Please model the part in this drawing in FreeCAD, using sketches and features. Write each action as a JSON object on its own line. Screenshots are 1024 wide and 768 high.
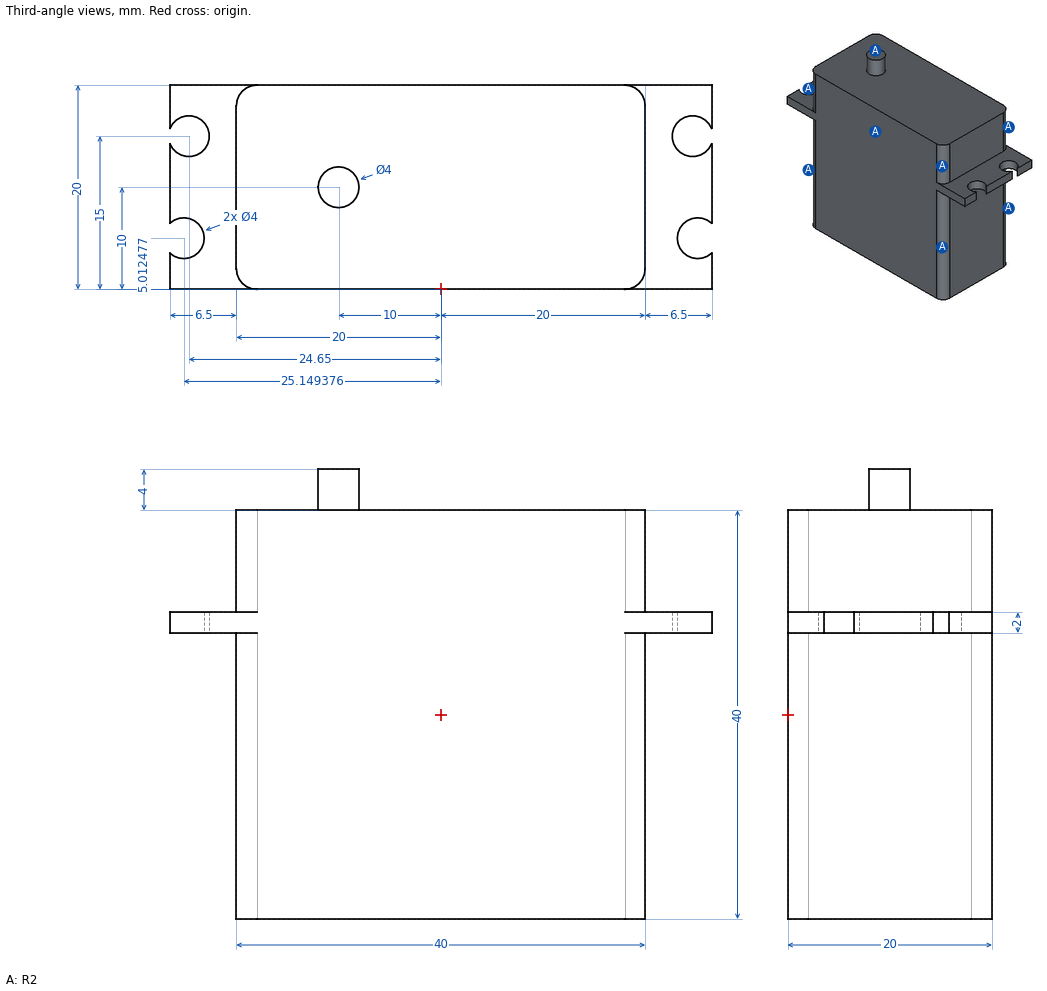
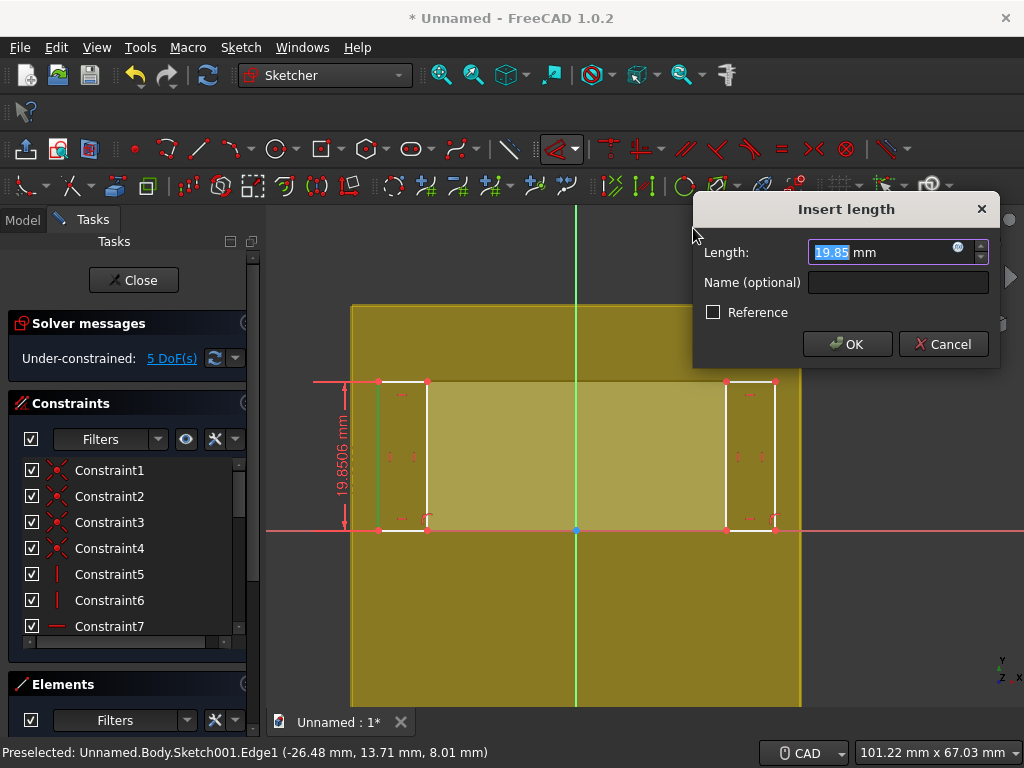
{"action": "type", "text": "20"}
{"action": "key", "text": "Return"}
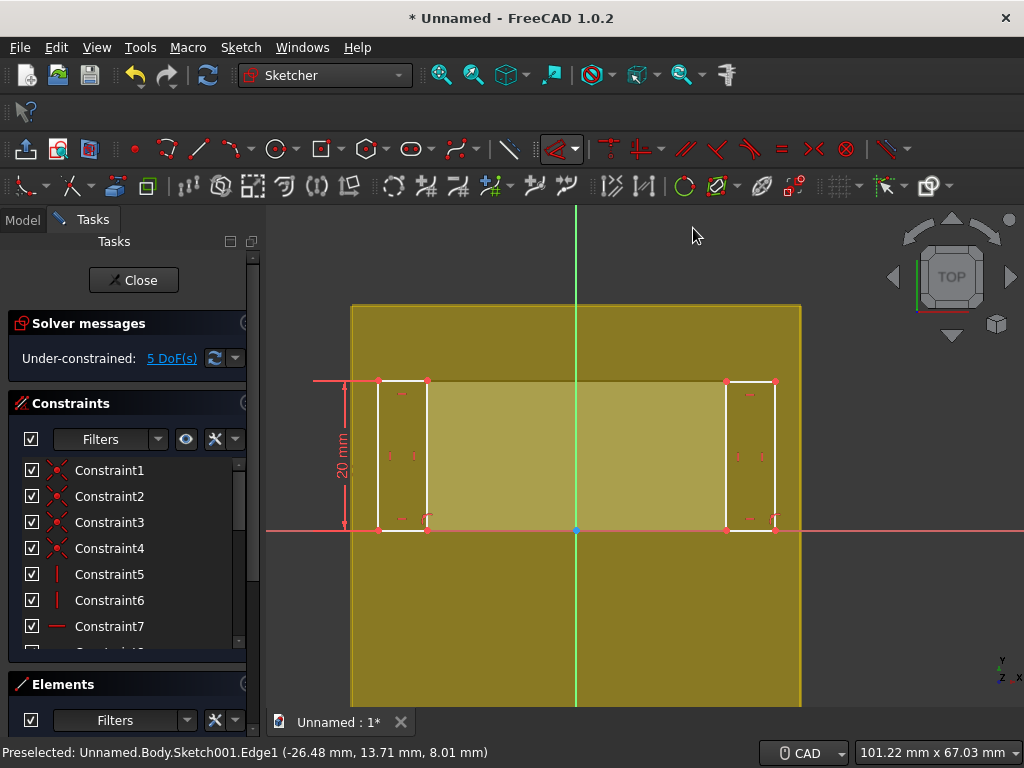
{"action": "left_click", "coordinate": [726, 427]}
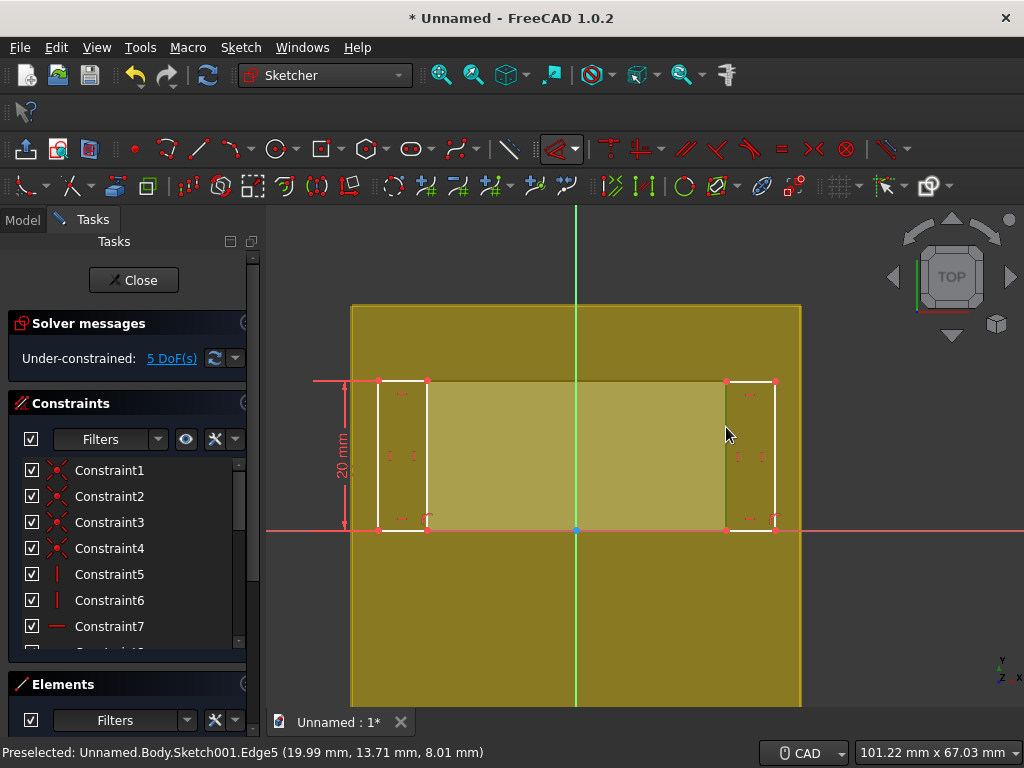
{"action": "key", "text": "i"}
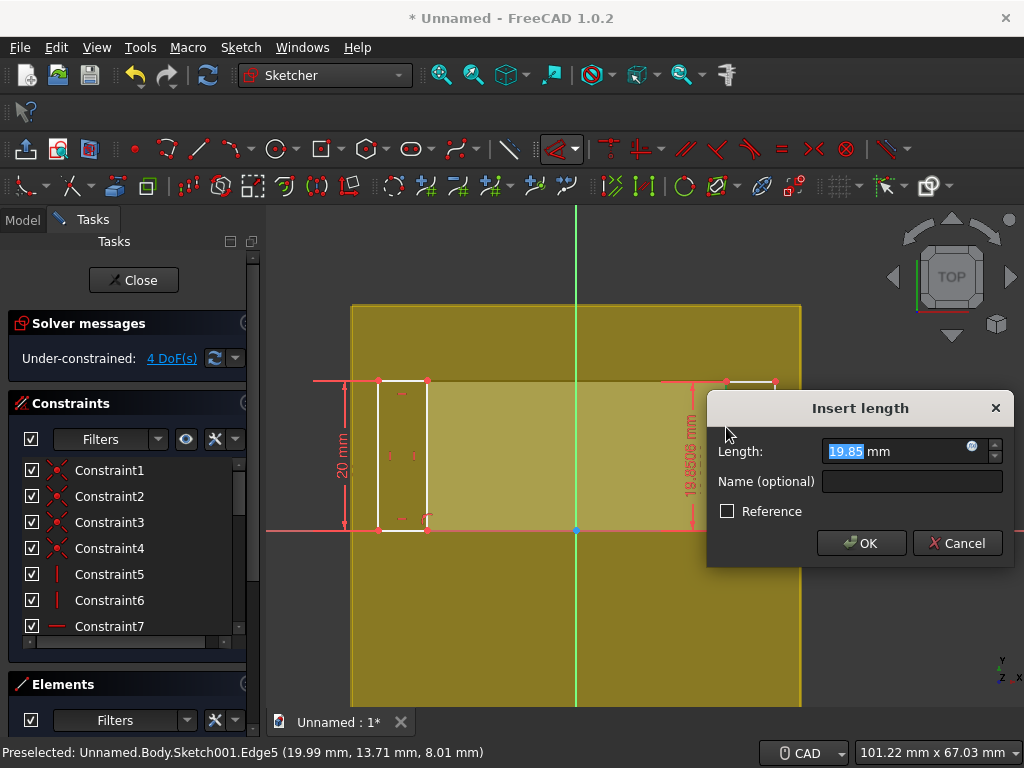
{"action": "type", "text": "20"}
{"action": "key", "text": "Return"}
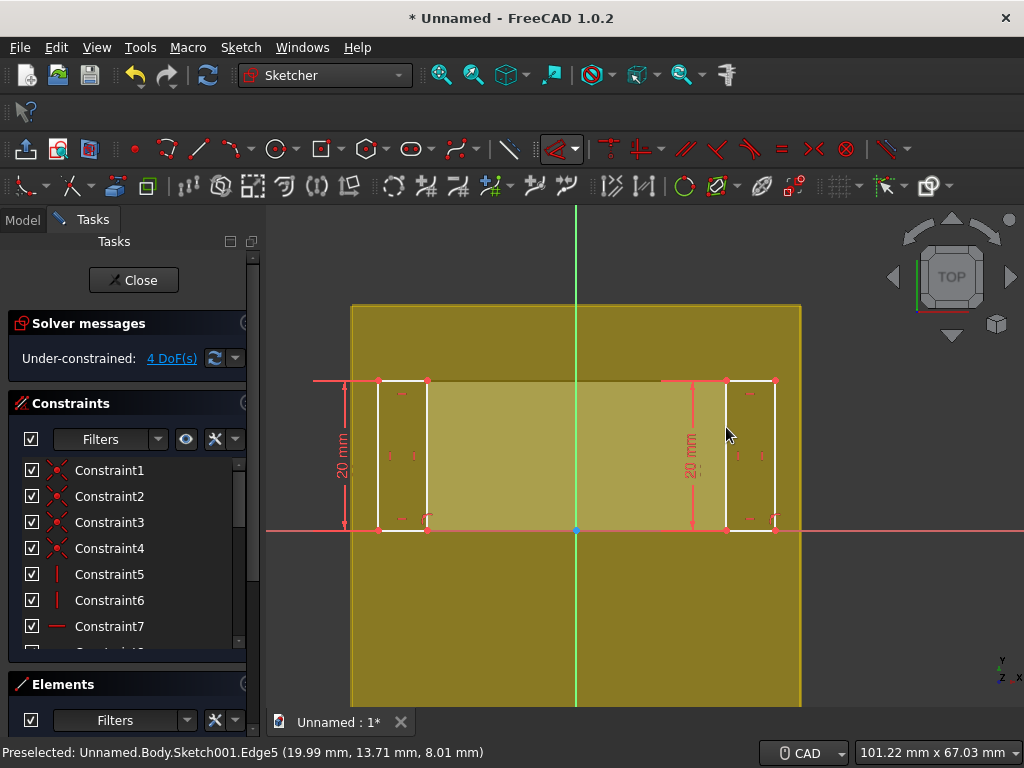
{"action": "left_click", "coordinate": [393, 531]}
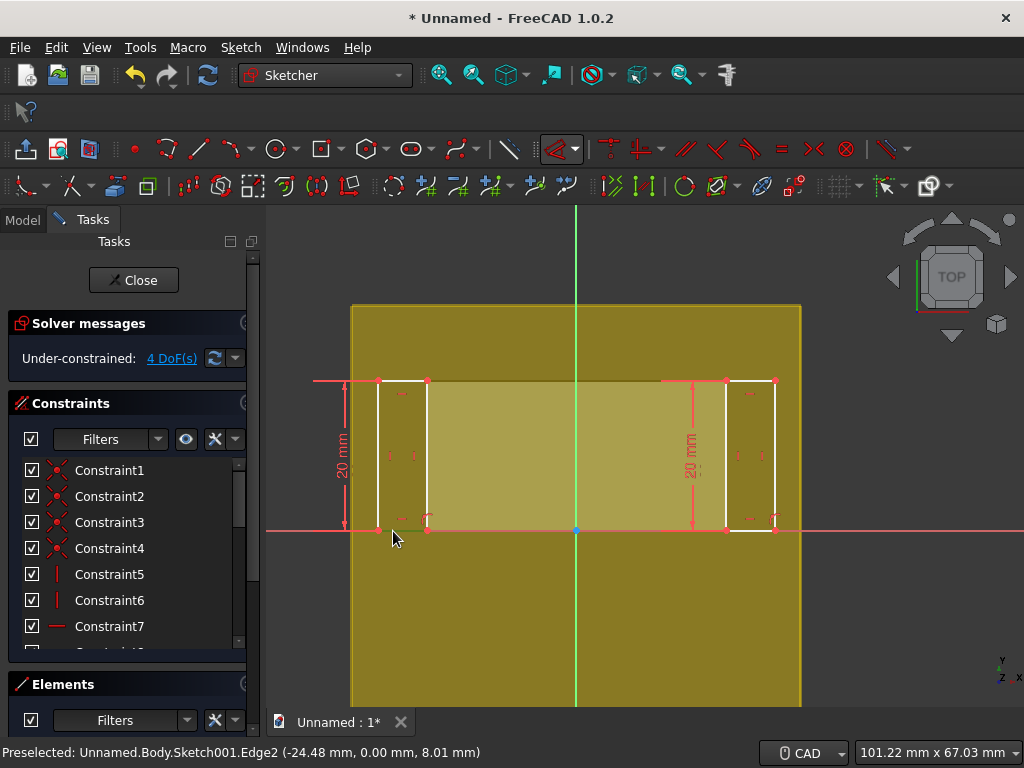
{"action": "key", "text": "l"}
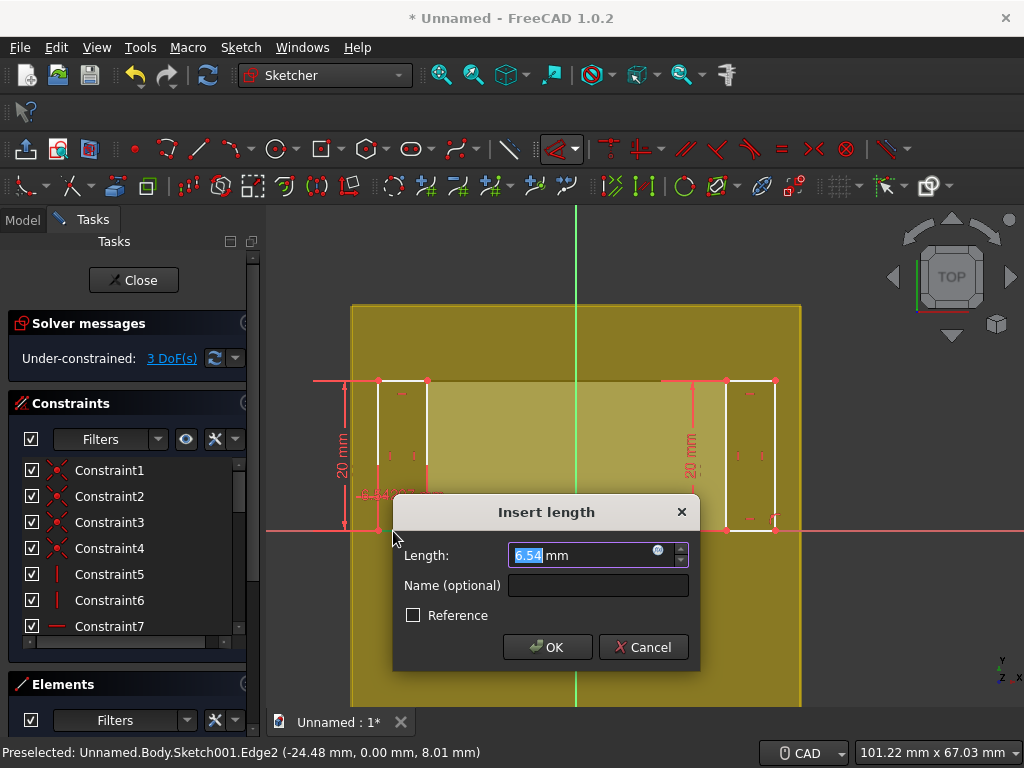
{"action": "type", "text": "6.5"}
{"action": "key", "text": "Return"}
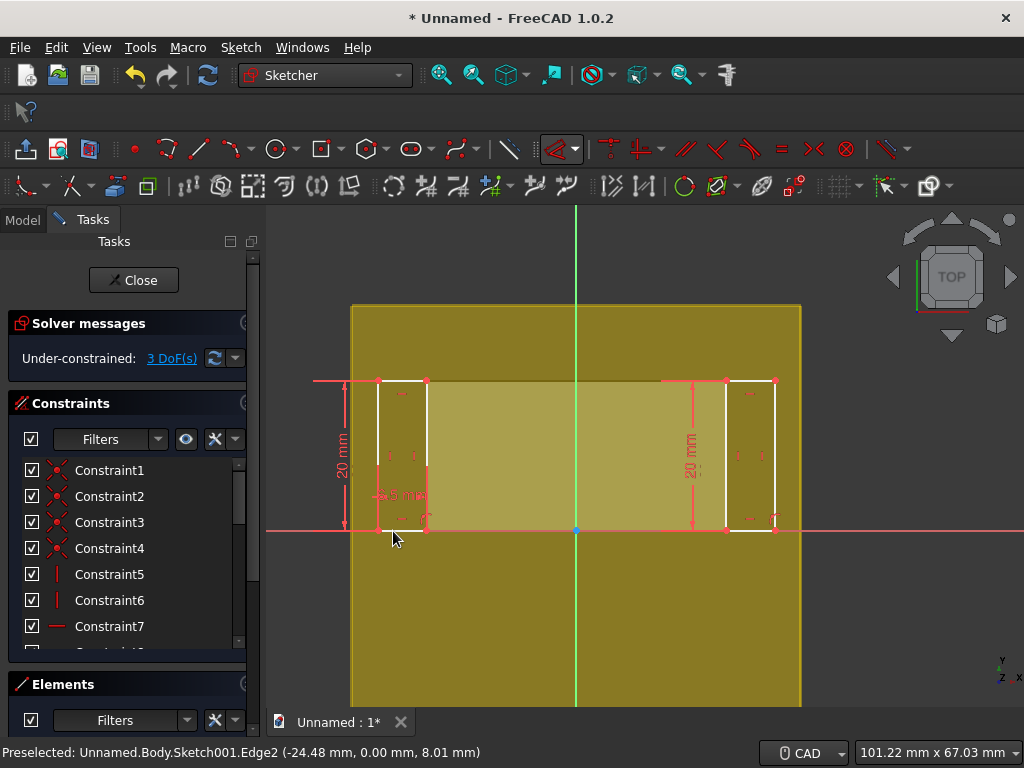
{"action": "left_click", "coordinate": [741, 531]}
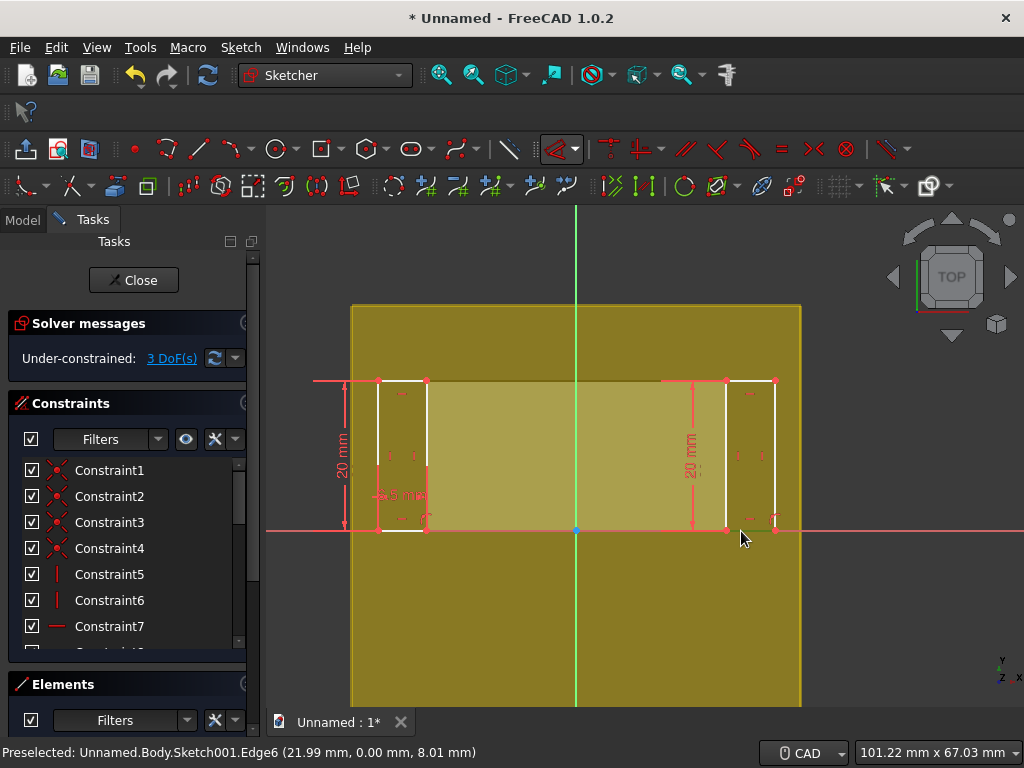
{"action": "key", "text": "l"}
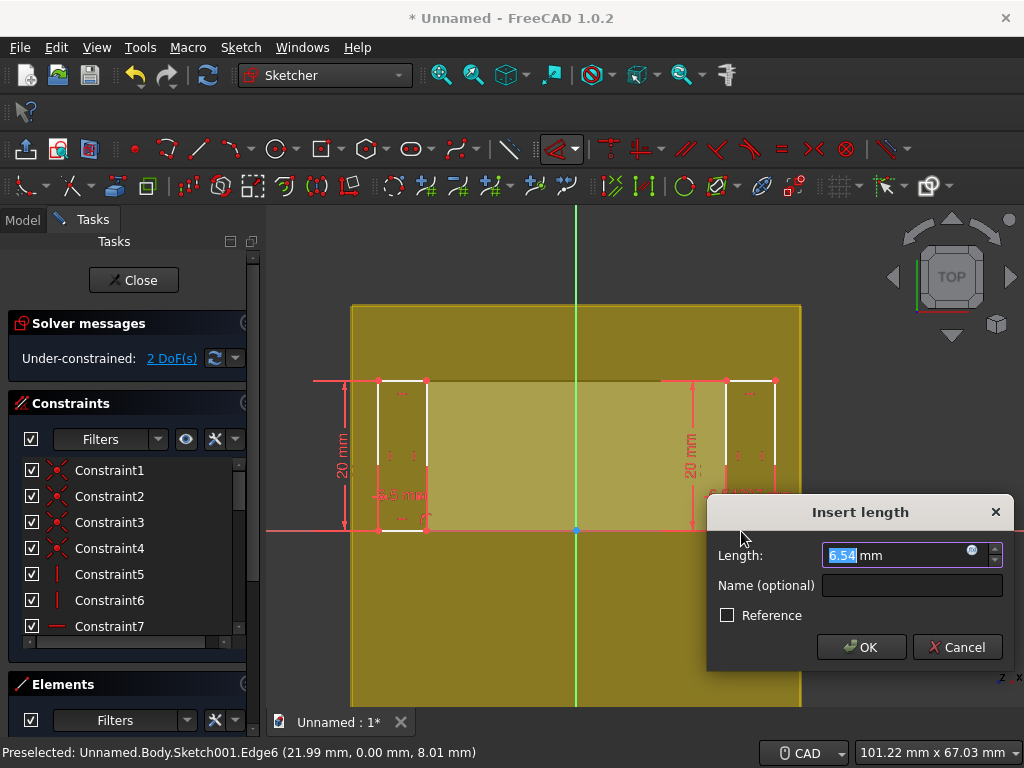
{"action": "type", "text": "6.5"}
{"action": "key", "text": "Return"}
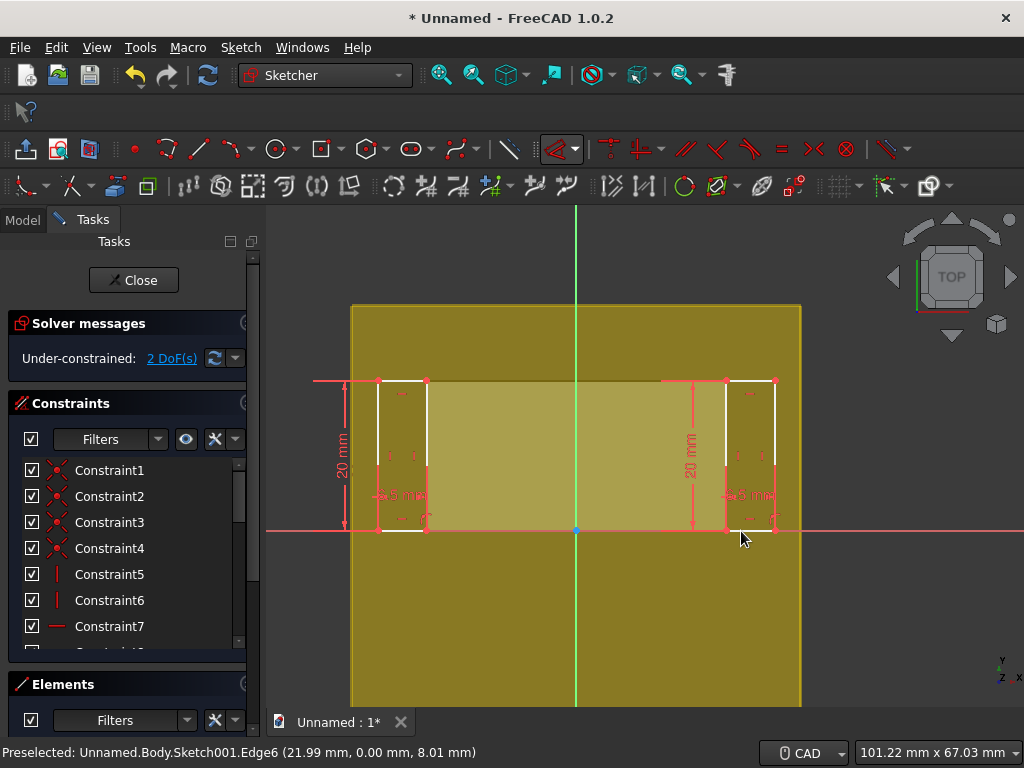
{"action": "left_click", "coordinate": [427, 531]}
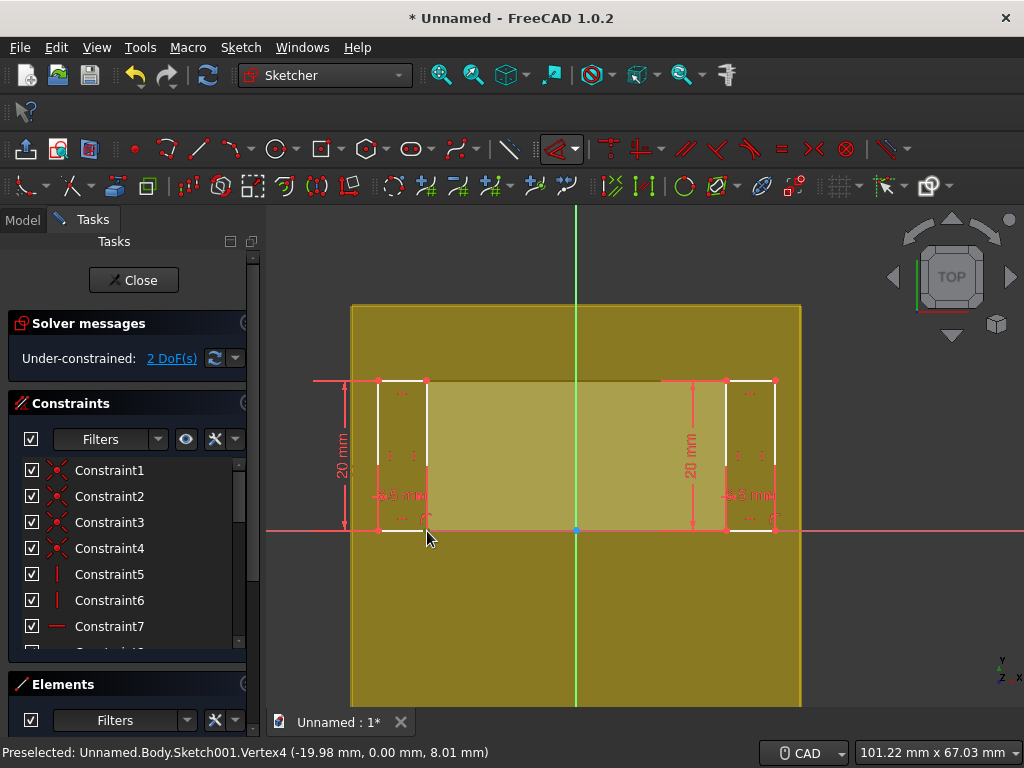
{"action": "key", "text": "l"}